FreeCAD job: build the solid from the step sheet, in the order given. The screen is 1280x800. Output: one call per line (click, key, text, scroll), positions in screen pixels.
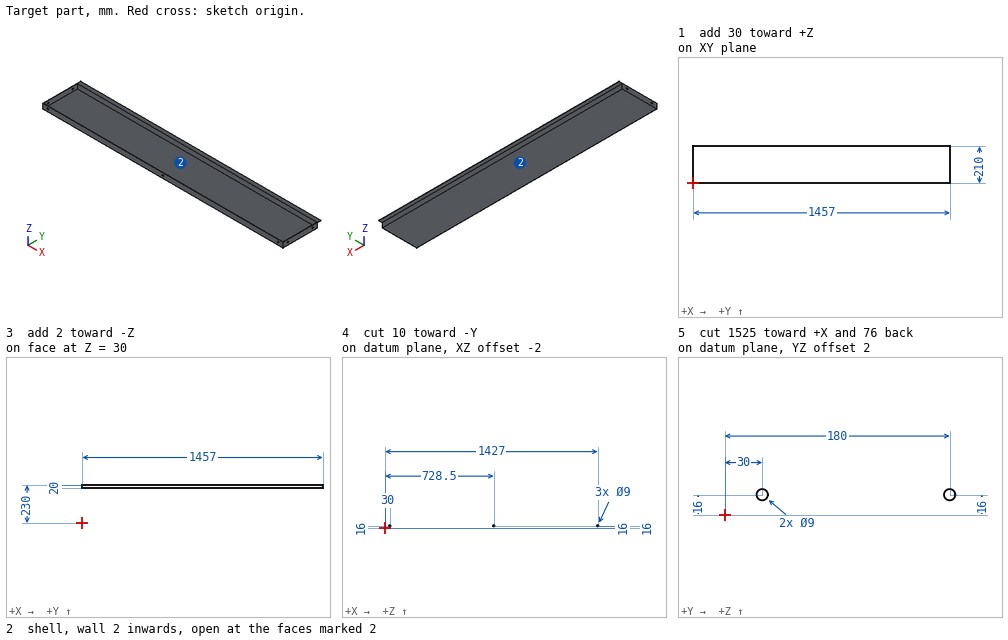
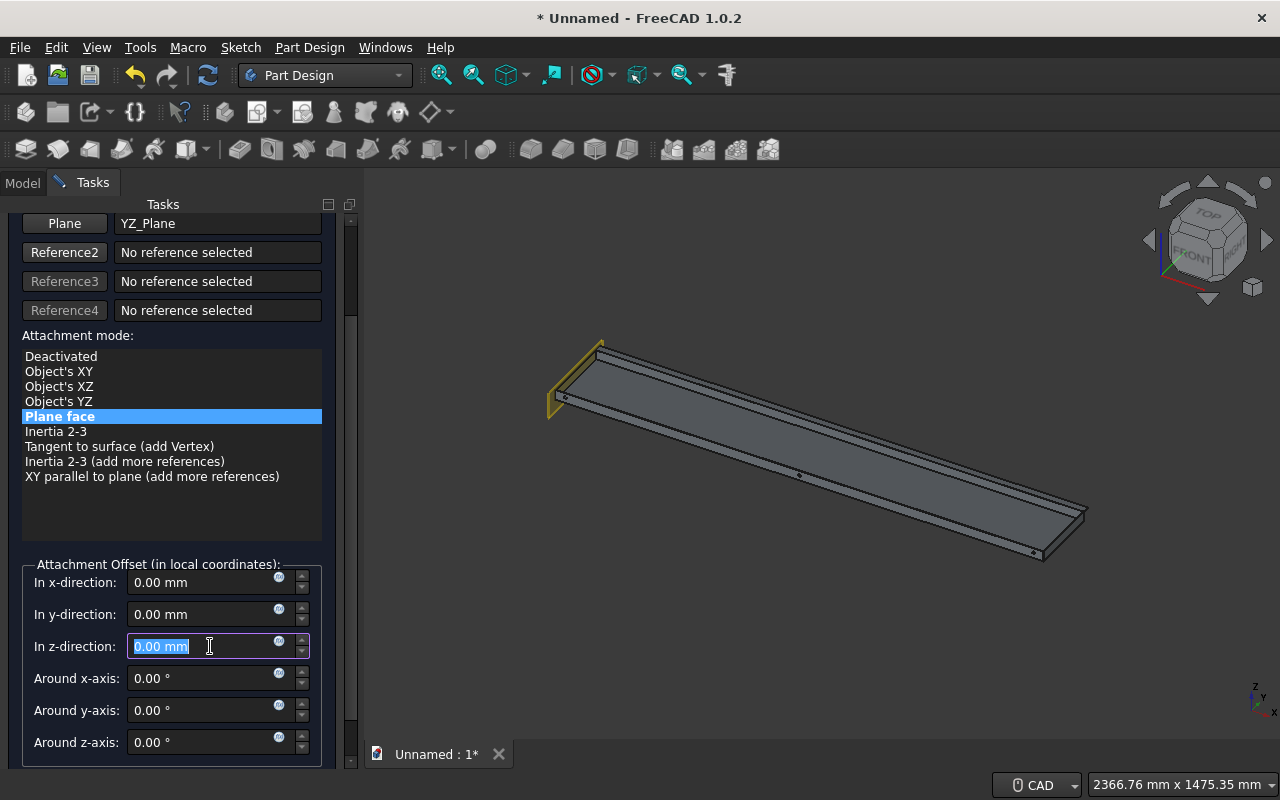
text(2)
key(Tab)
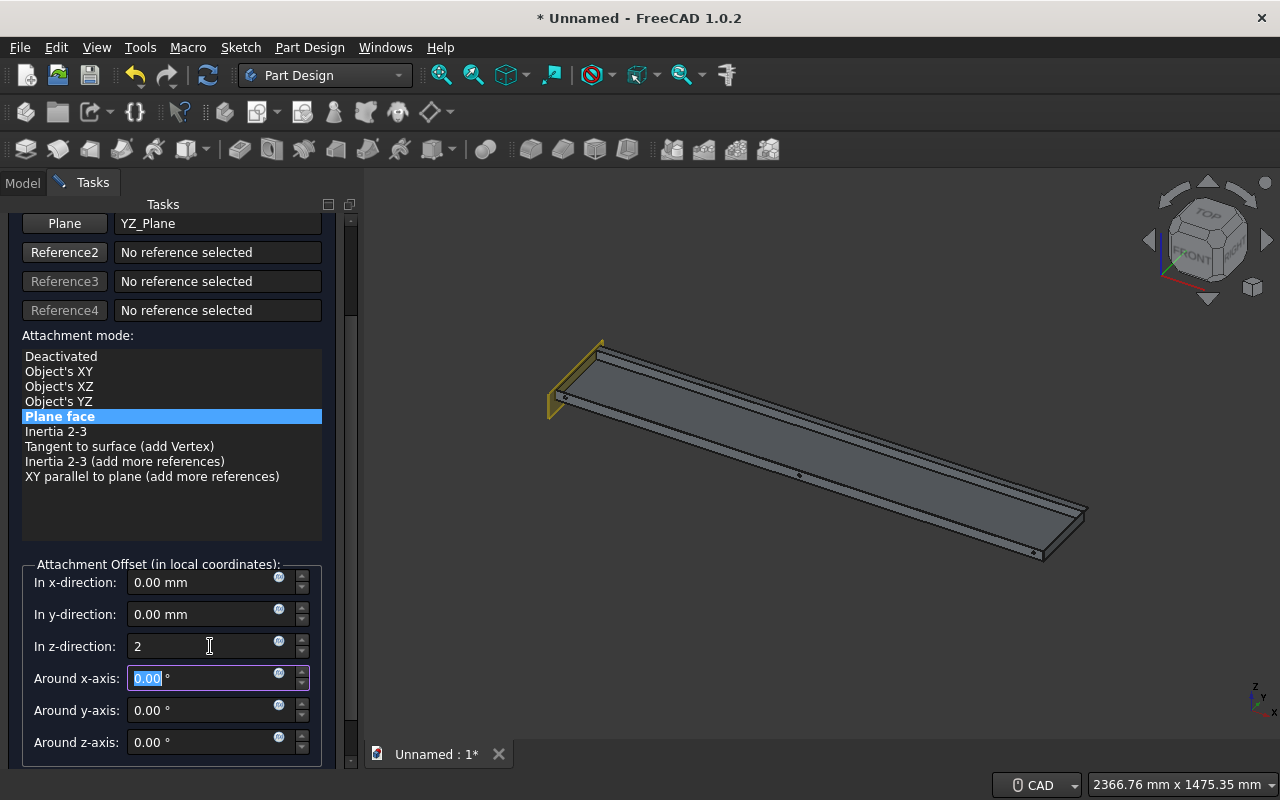
scroll(351, 491, up, 3)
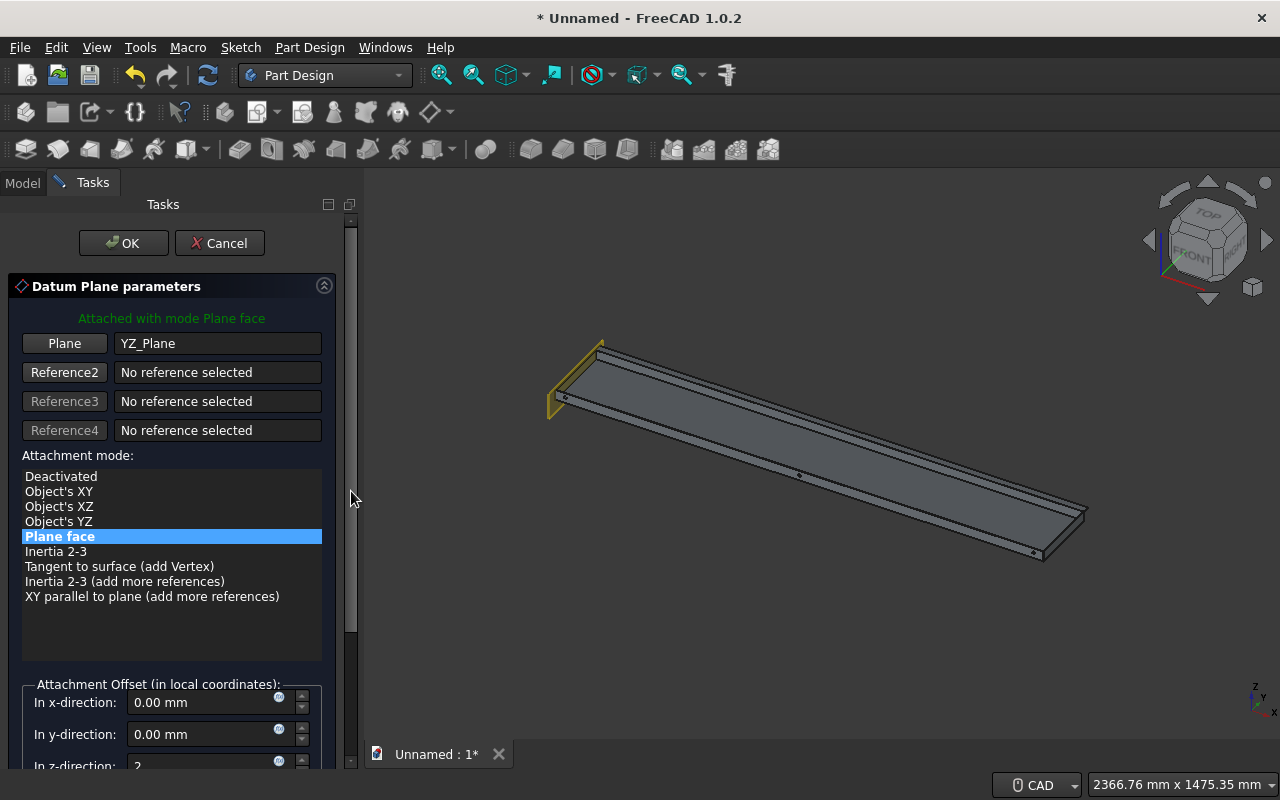
click(124, 243)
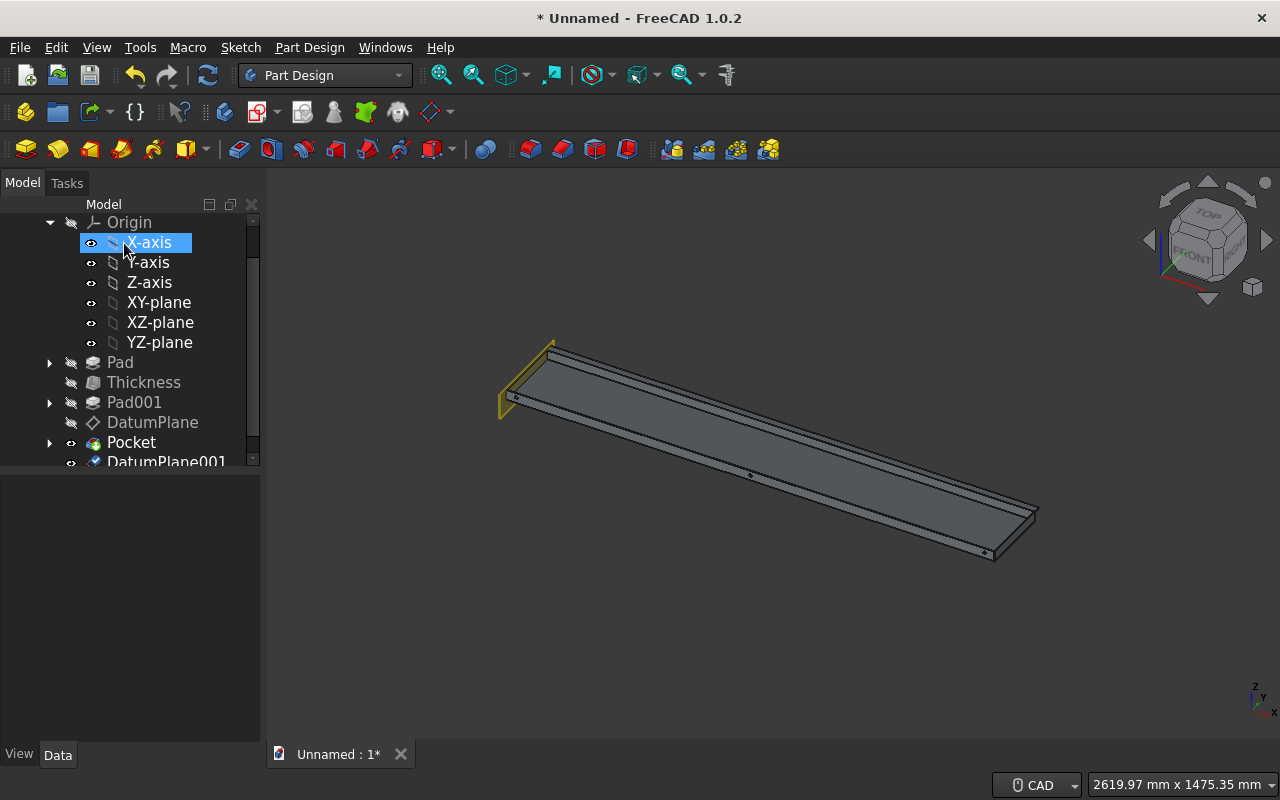
click(116, 463)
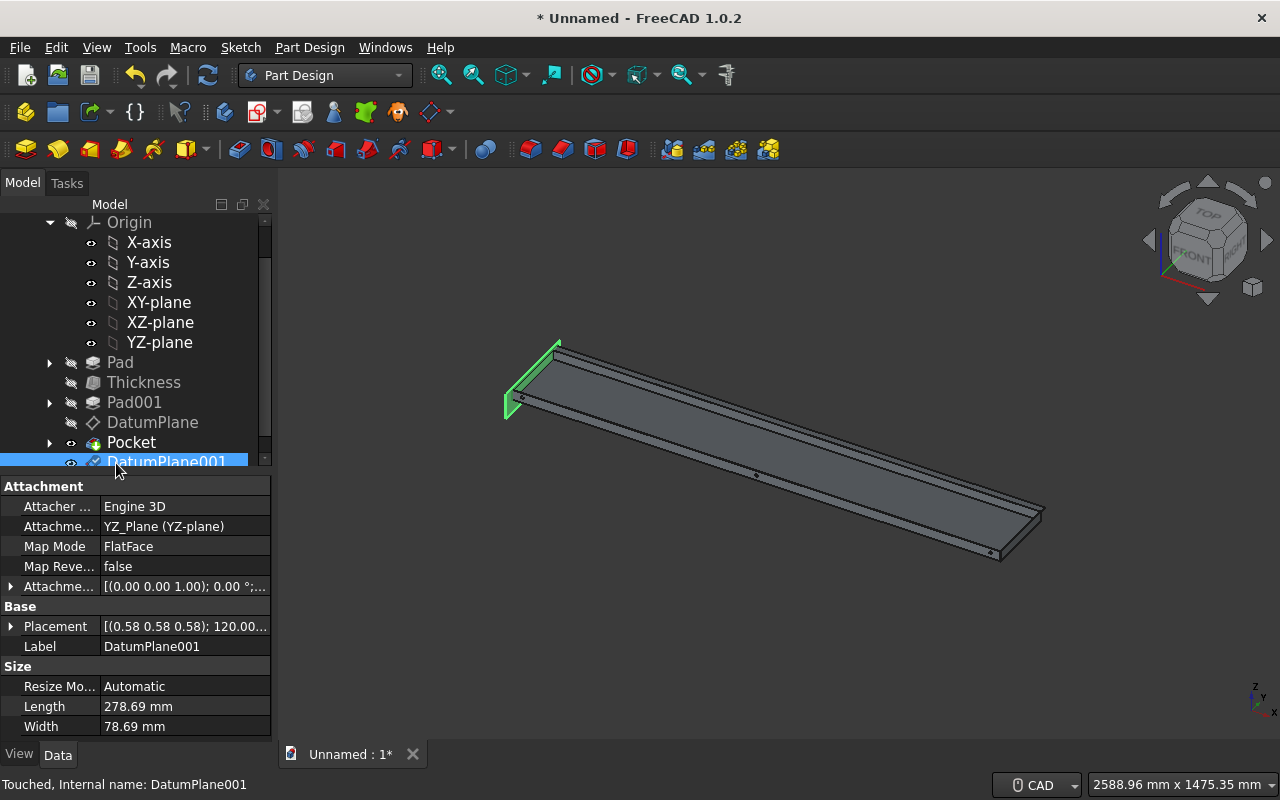
click(258, 112)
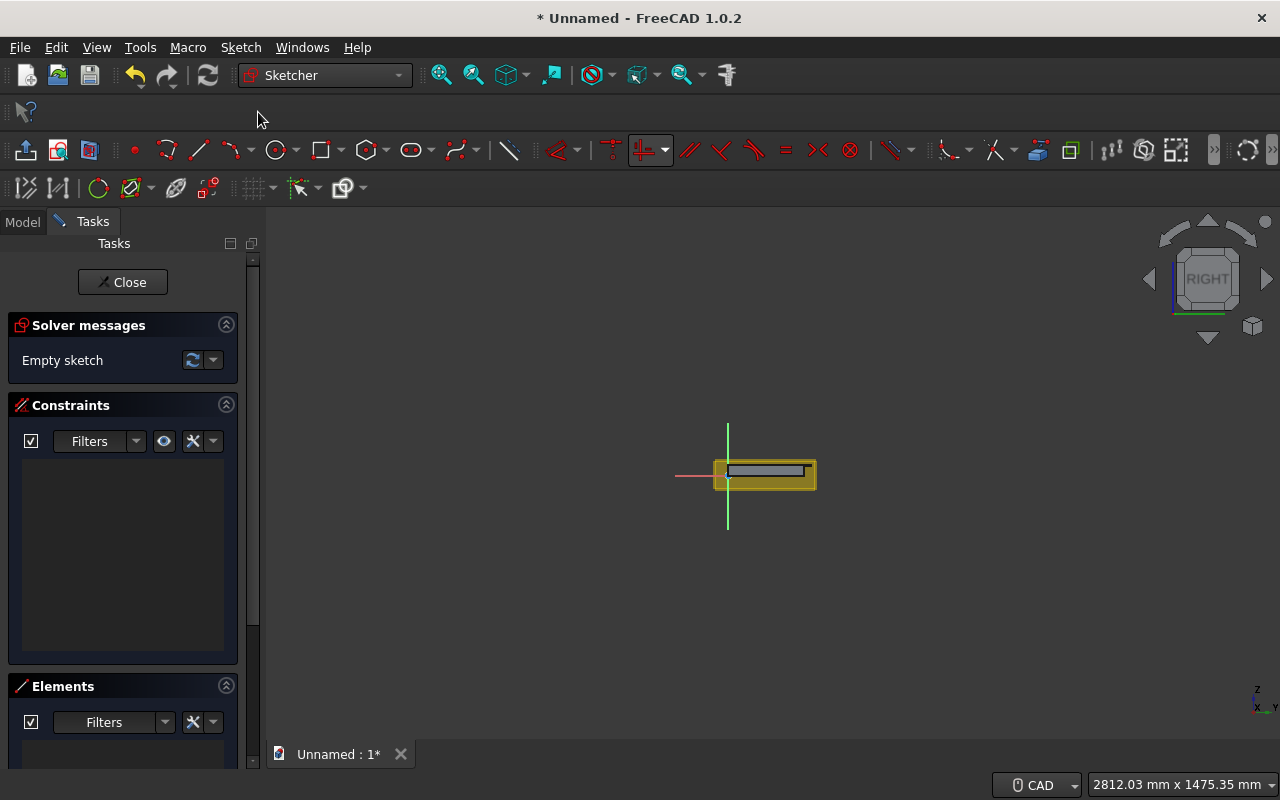
click(90, 150)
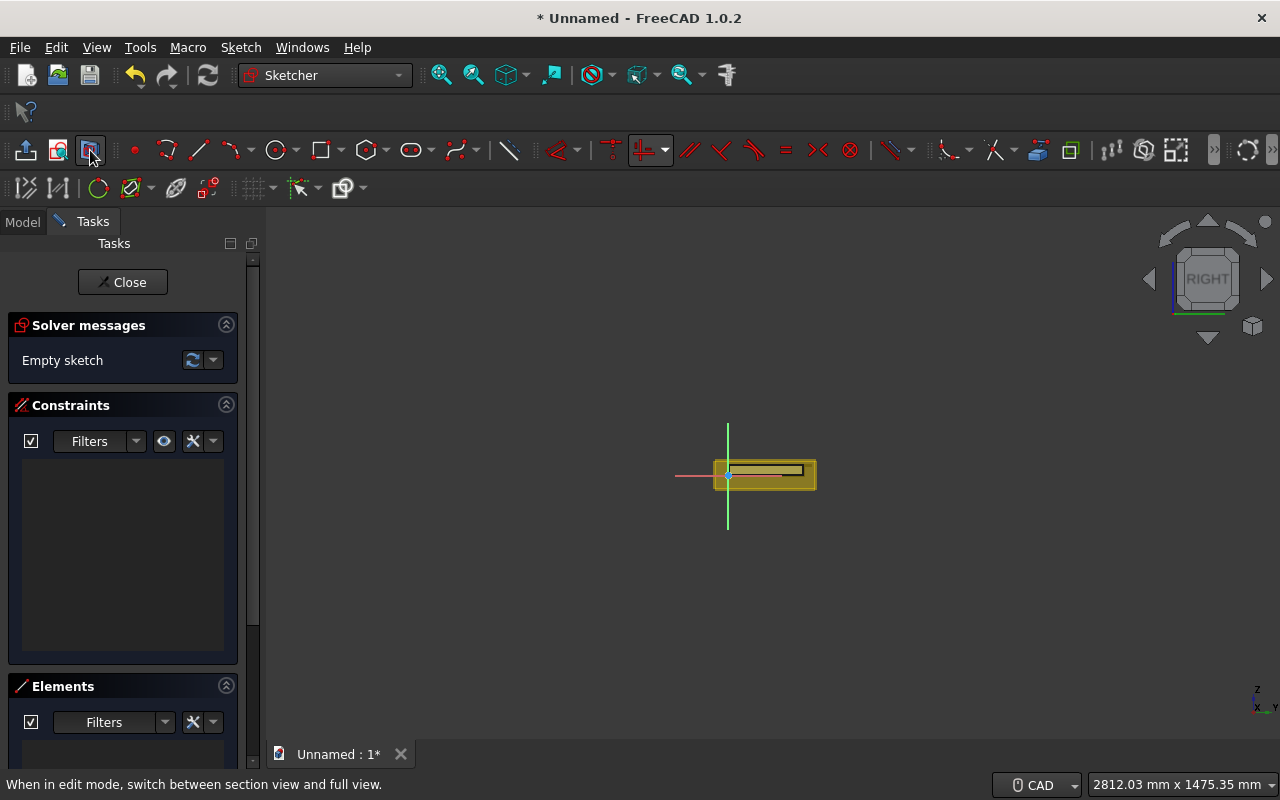
scroll(769, 472, up, 11)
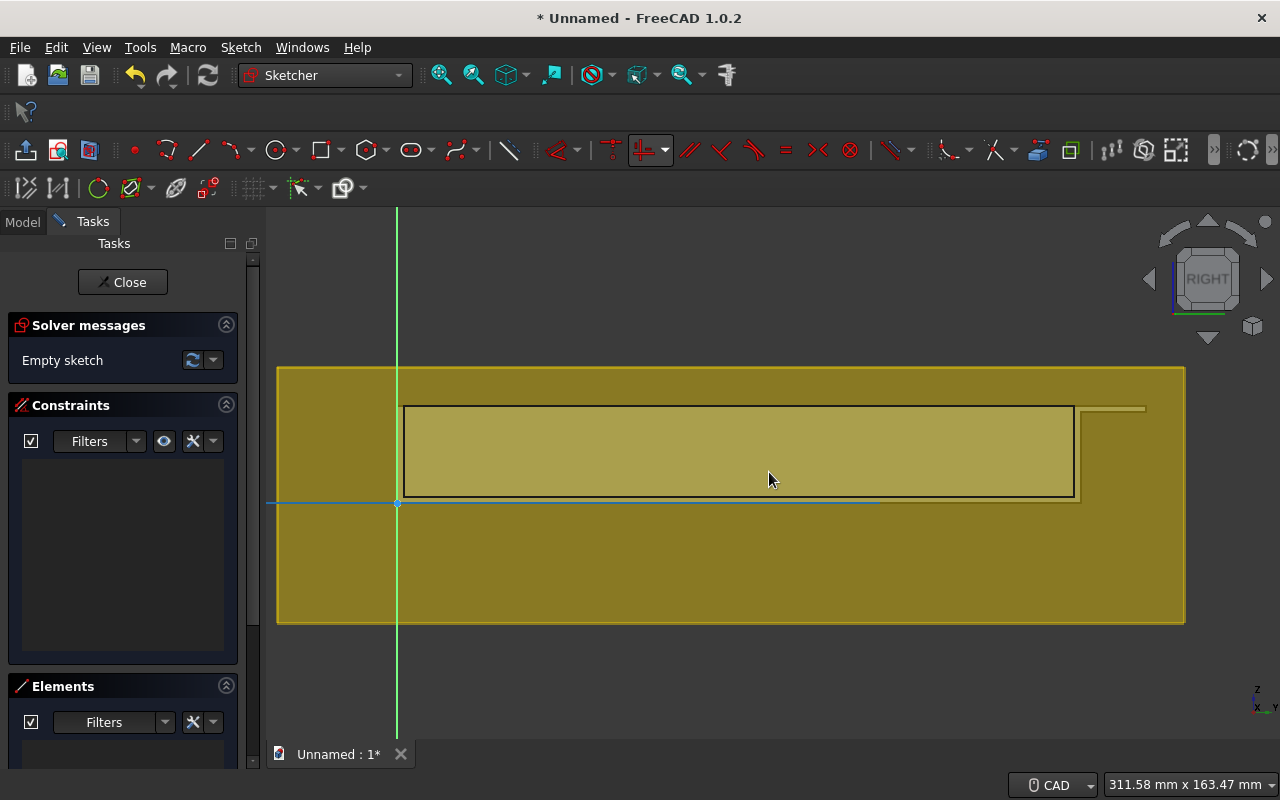
click(276, 150)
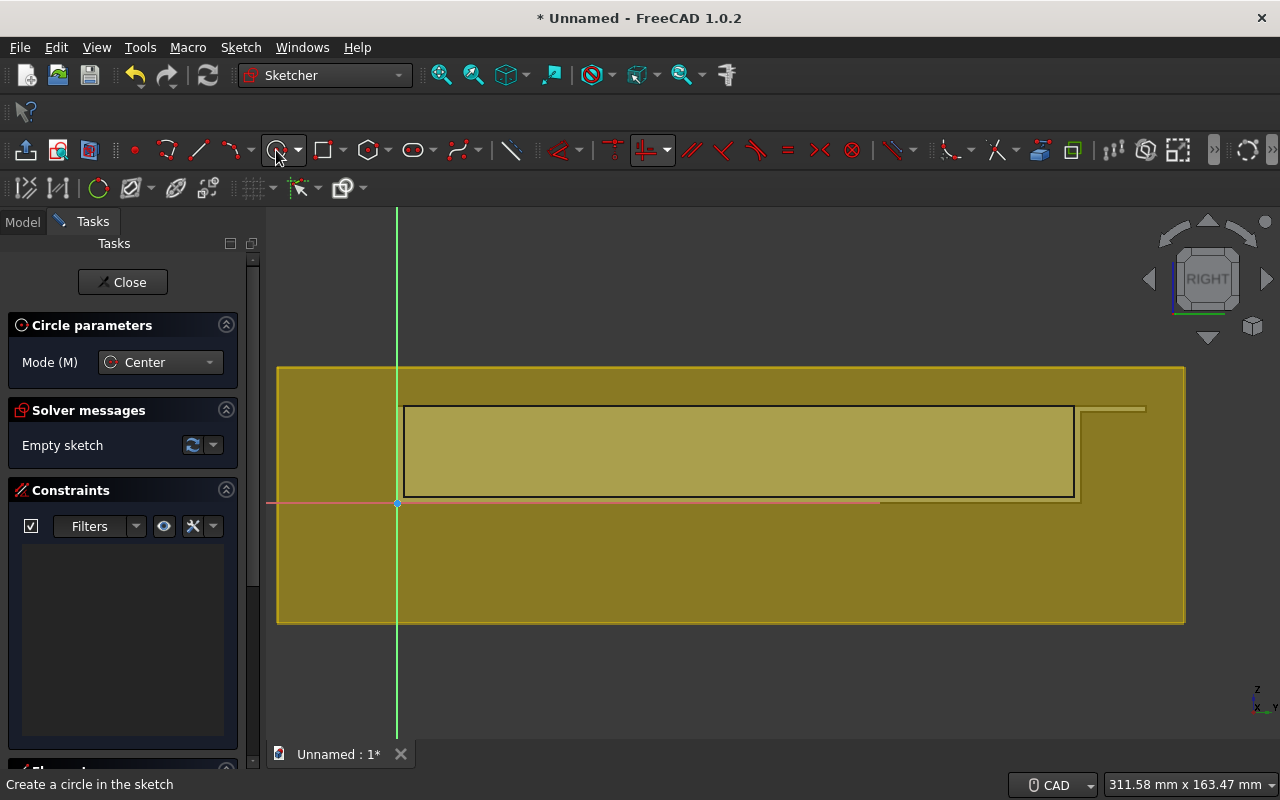
scroll(495, 451, up, 3)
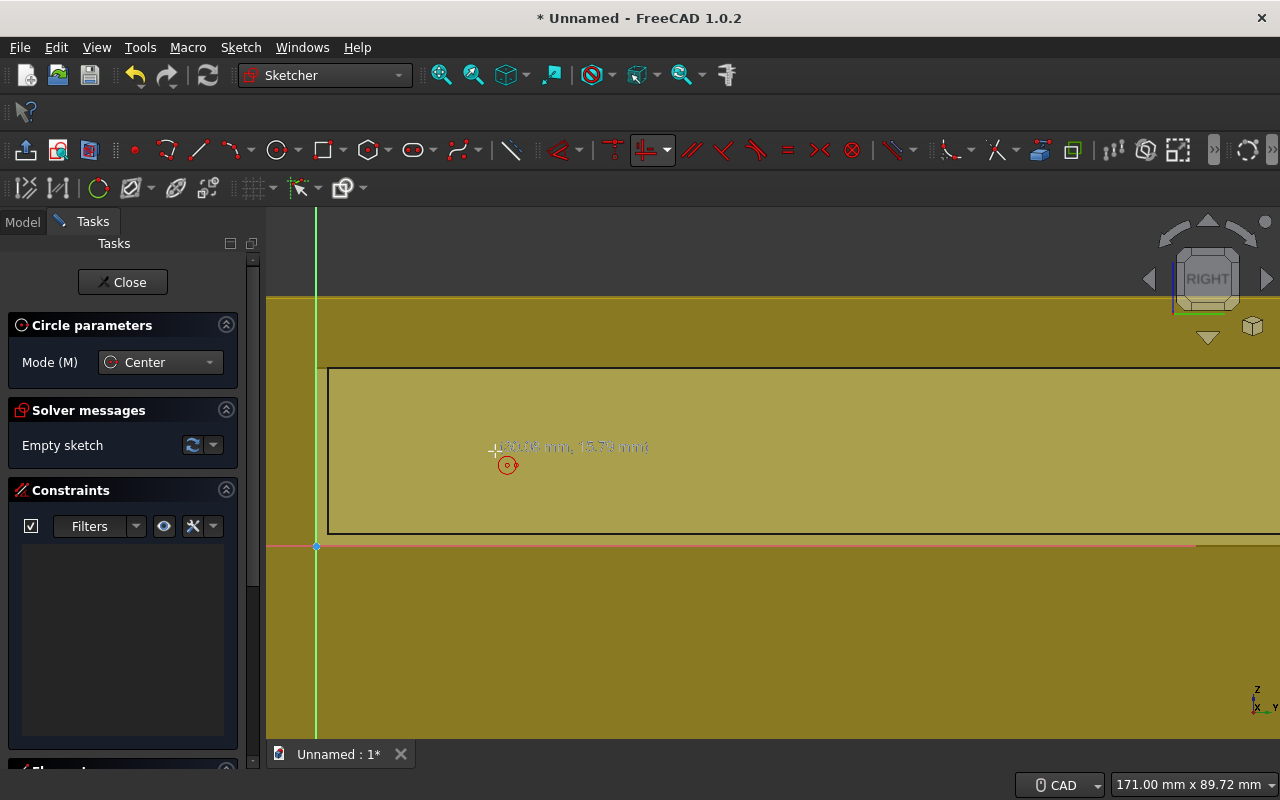
click(494, 451)
move(513, 432)